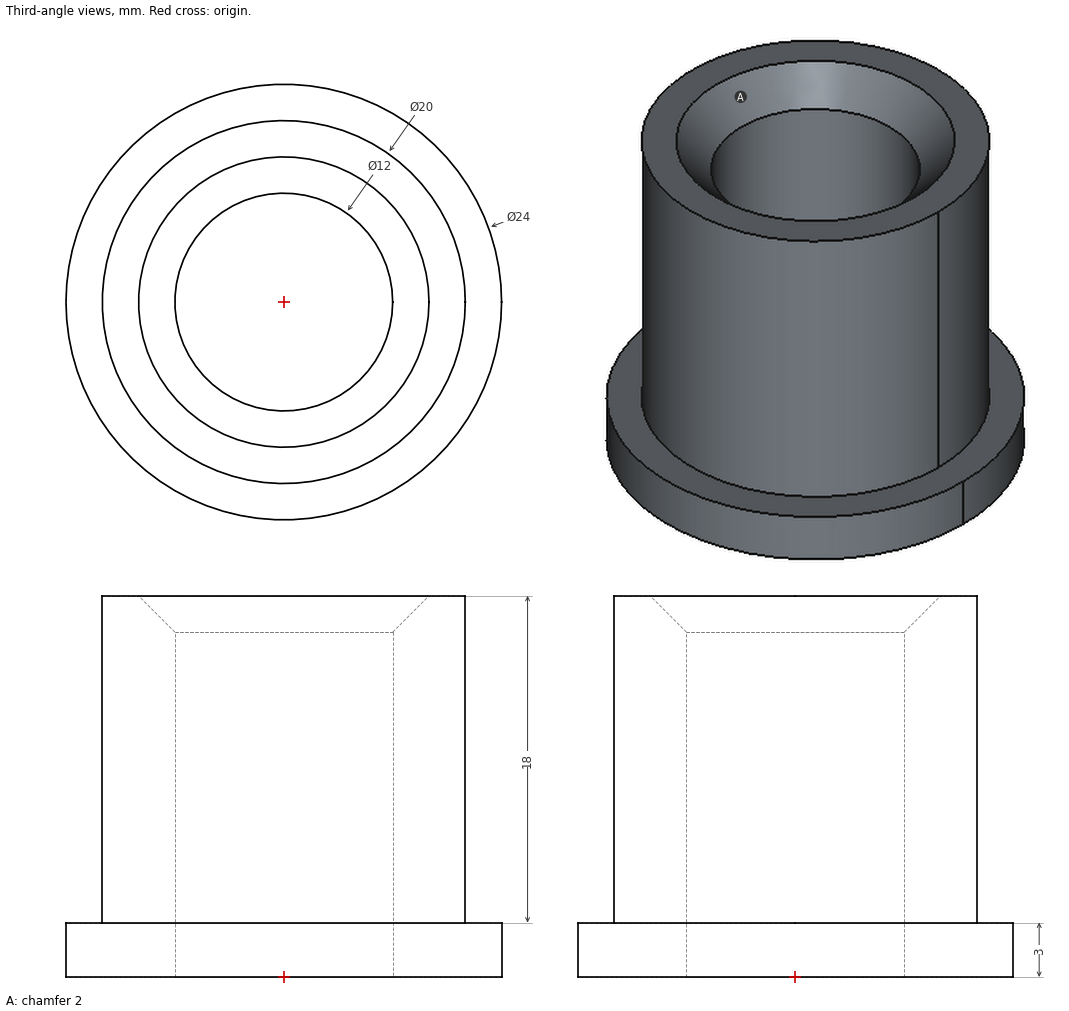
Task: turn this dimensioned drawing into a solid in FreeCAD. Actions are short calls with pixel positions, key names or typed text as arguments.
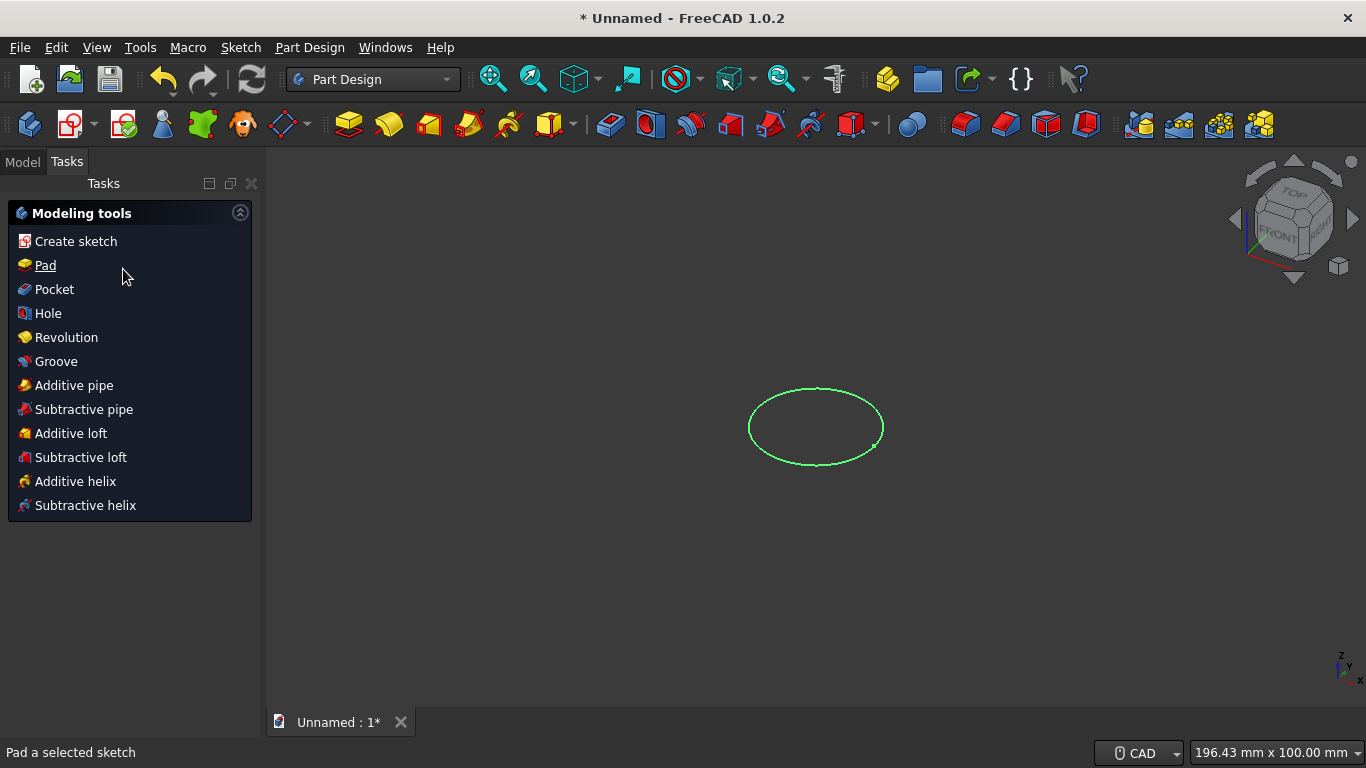
click(350, 124)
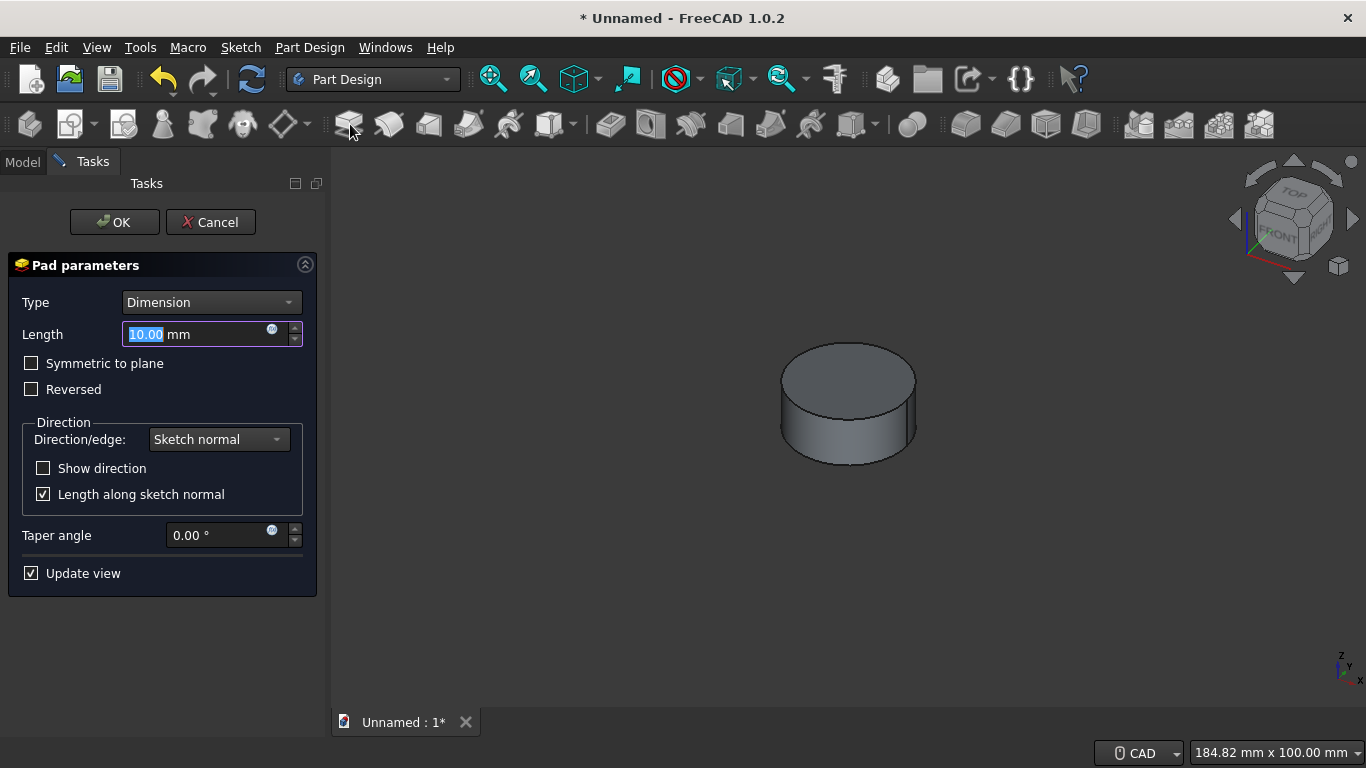
text(3)
key(Tab)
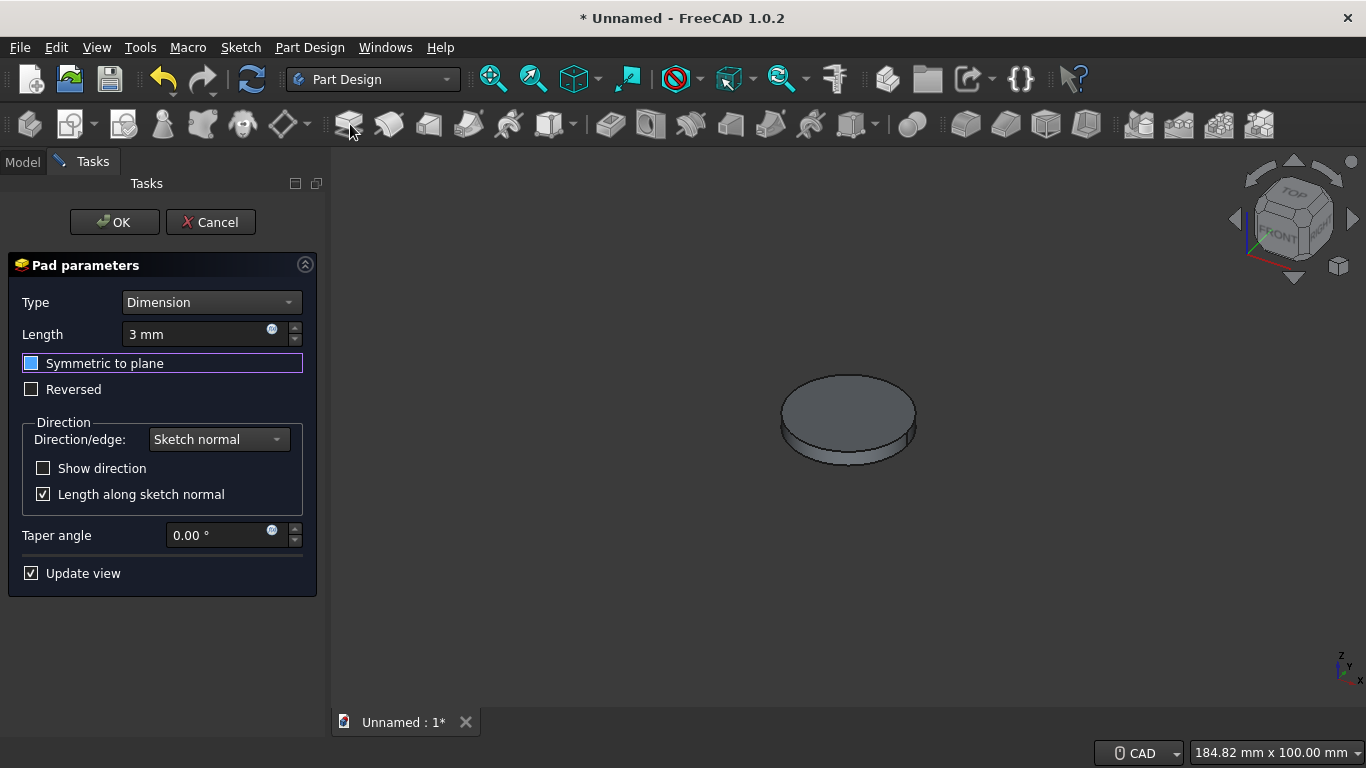
click(115, 222)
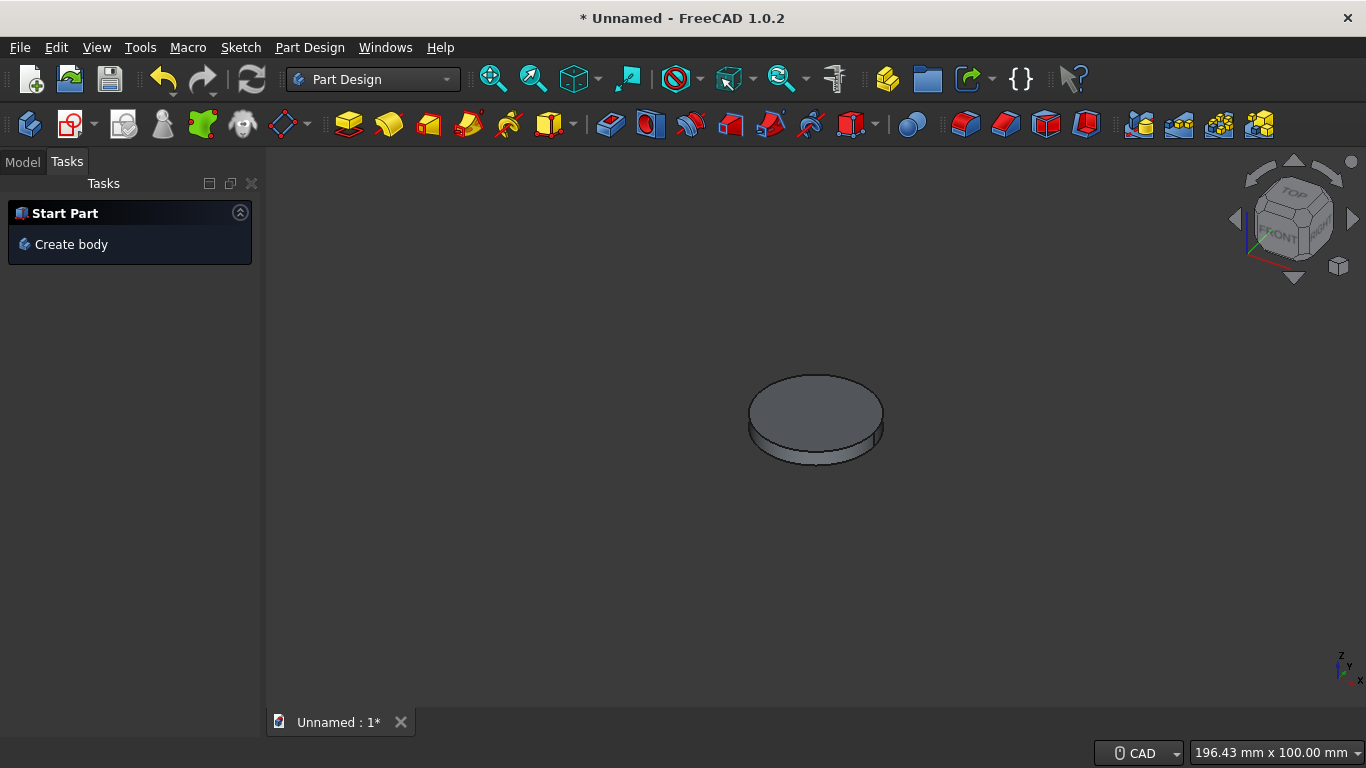
click(494, 80)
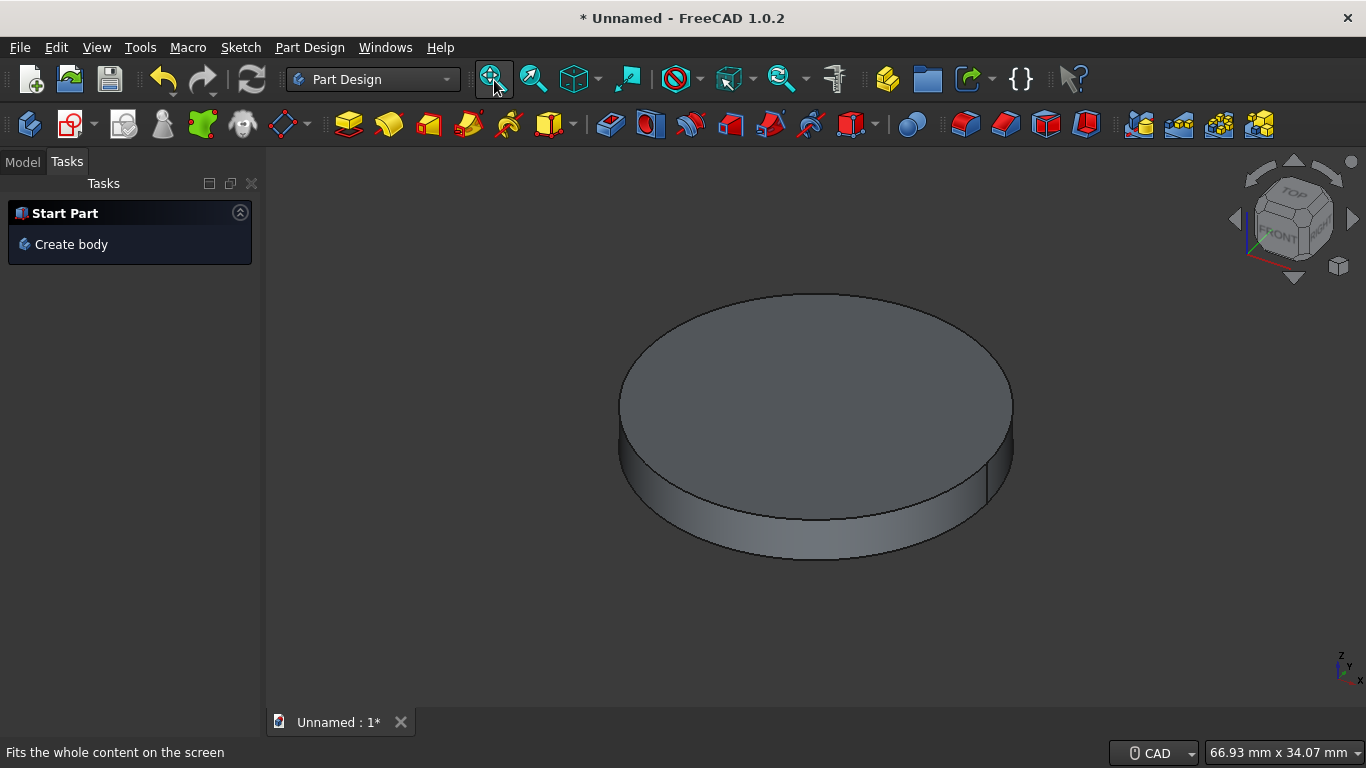
click(816, 406)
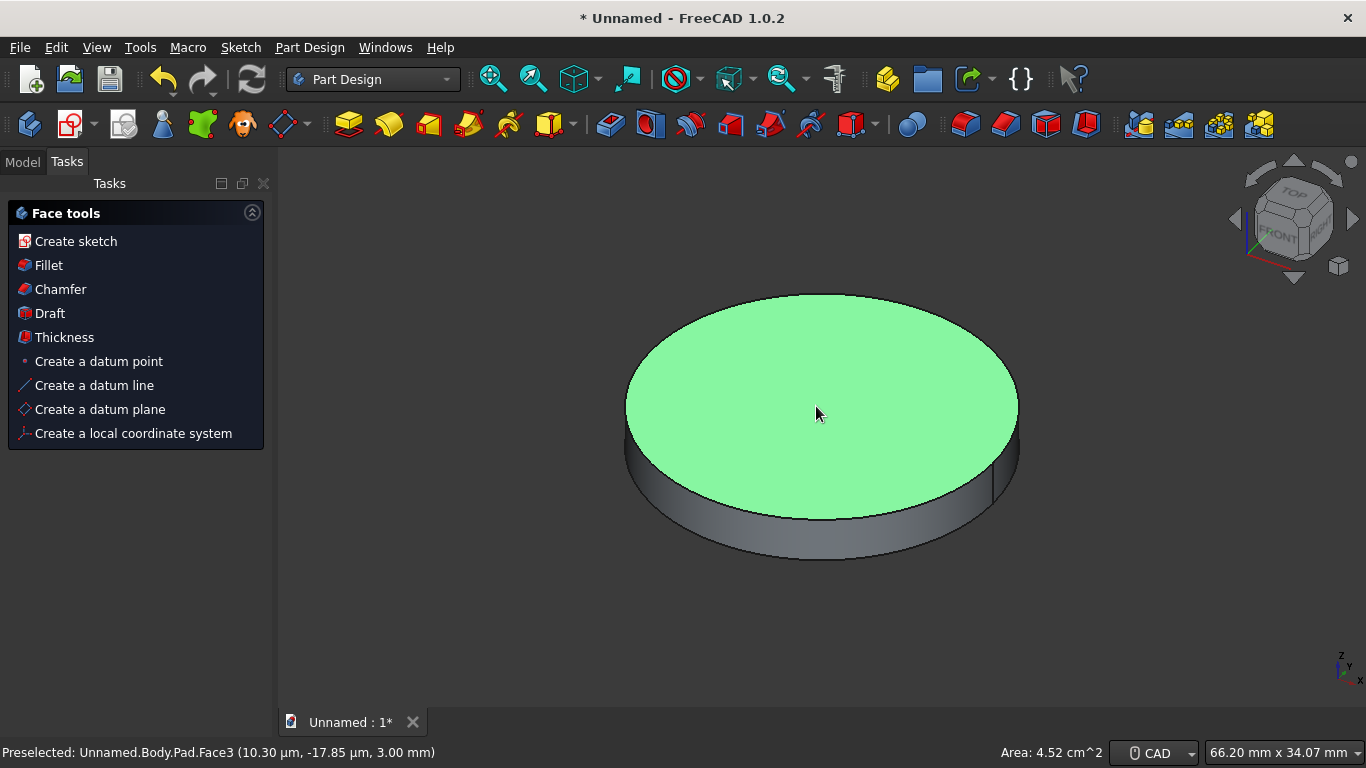
click(70, 124)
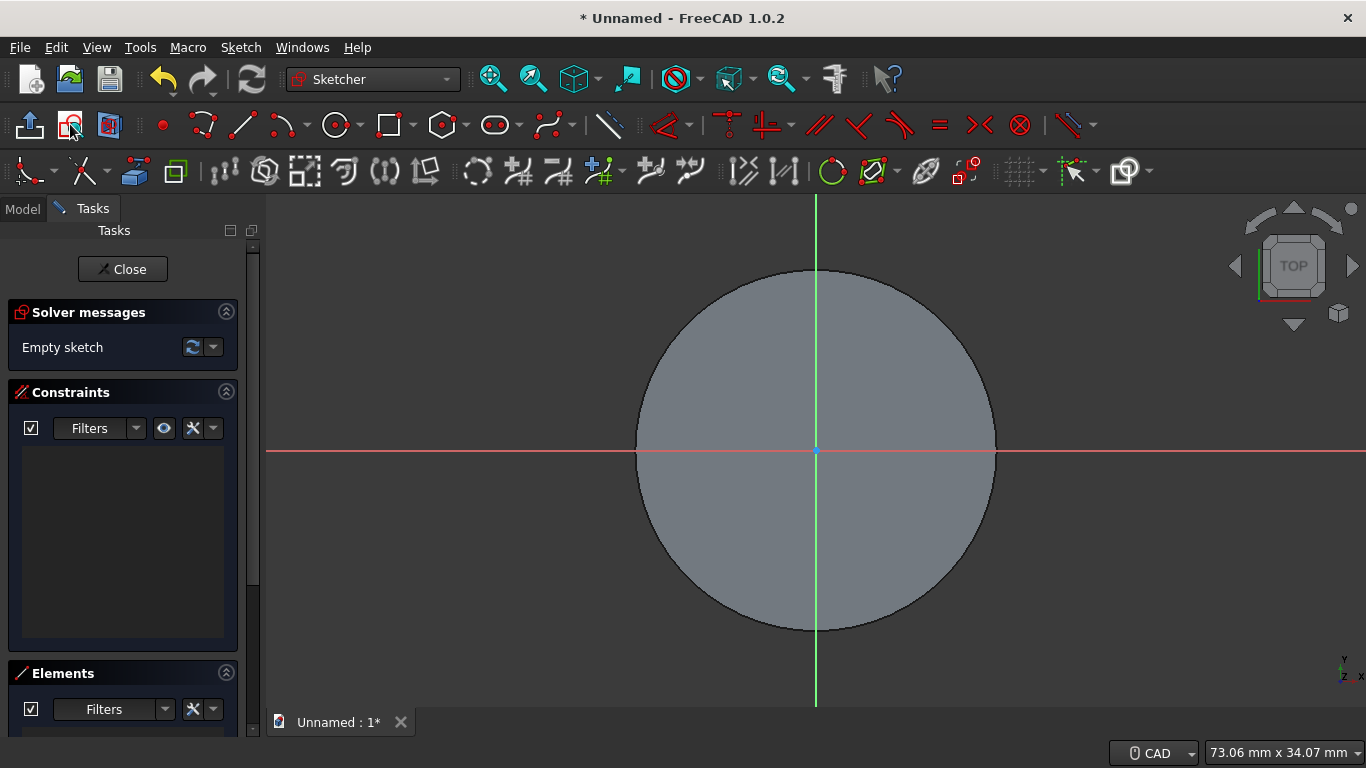
click(336, 126)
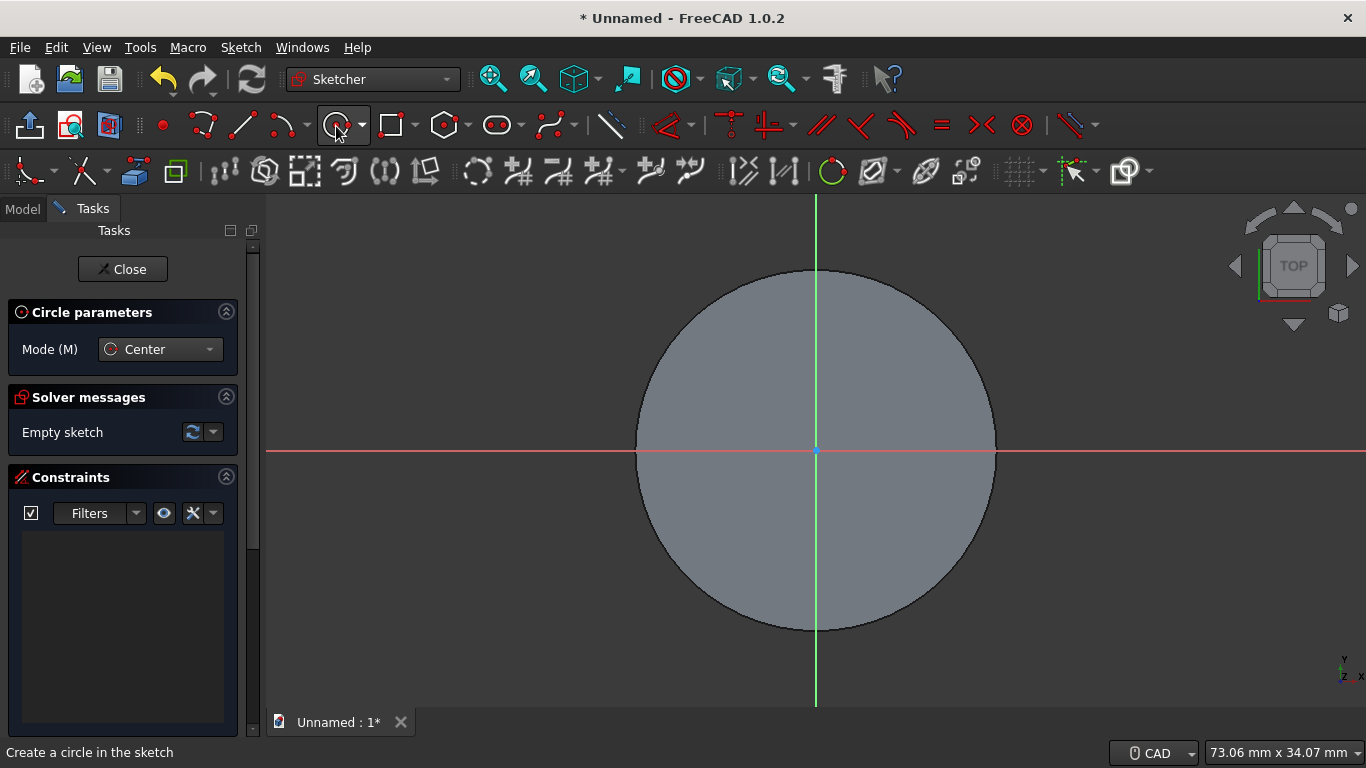
click(816, 450)
move(922, 344)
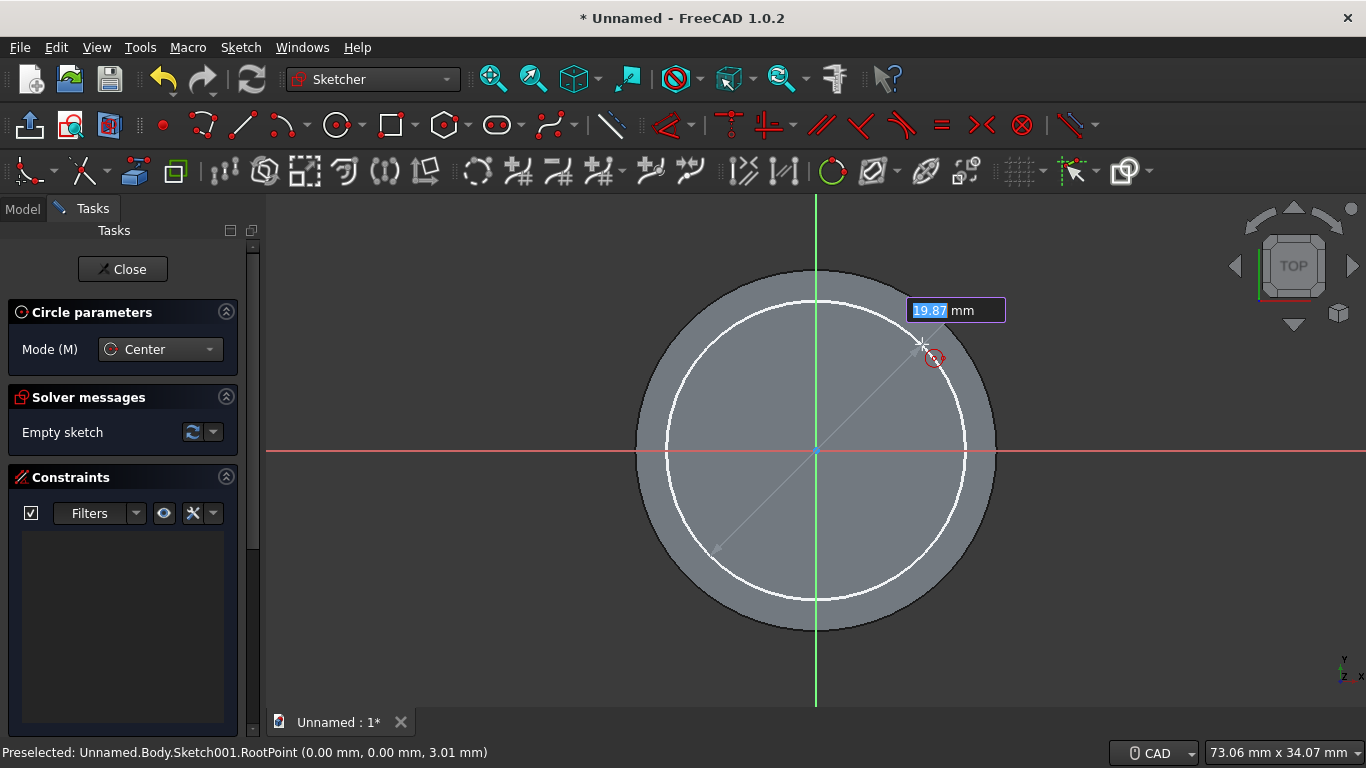
text(20)
key(Return)
key(Escape)